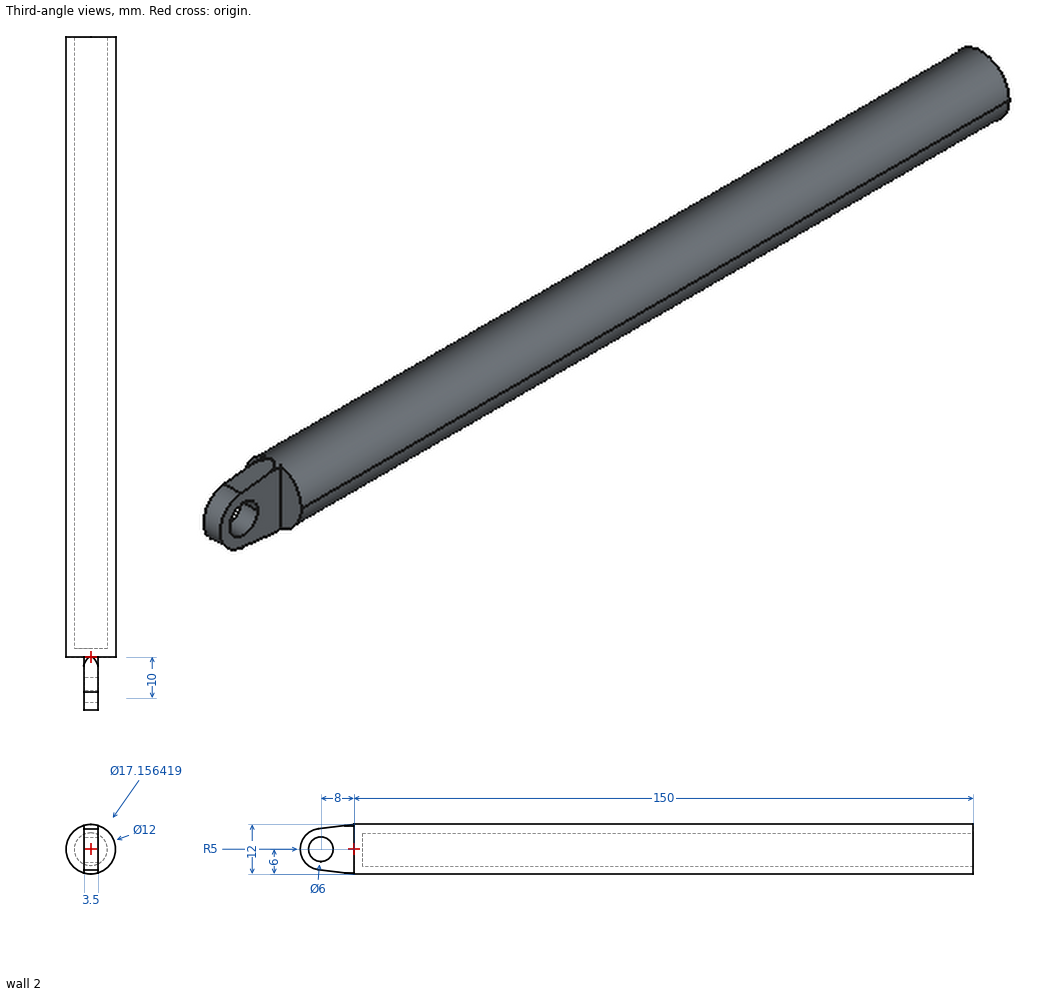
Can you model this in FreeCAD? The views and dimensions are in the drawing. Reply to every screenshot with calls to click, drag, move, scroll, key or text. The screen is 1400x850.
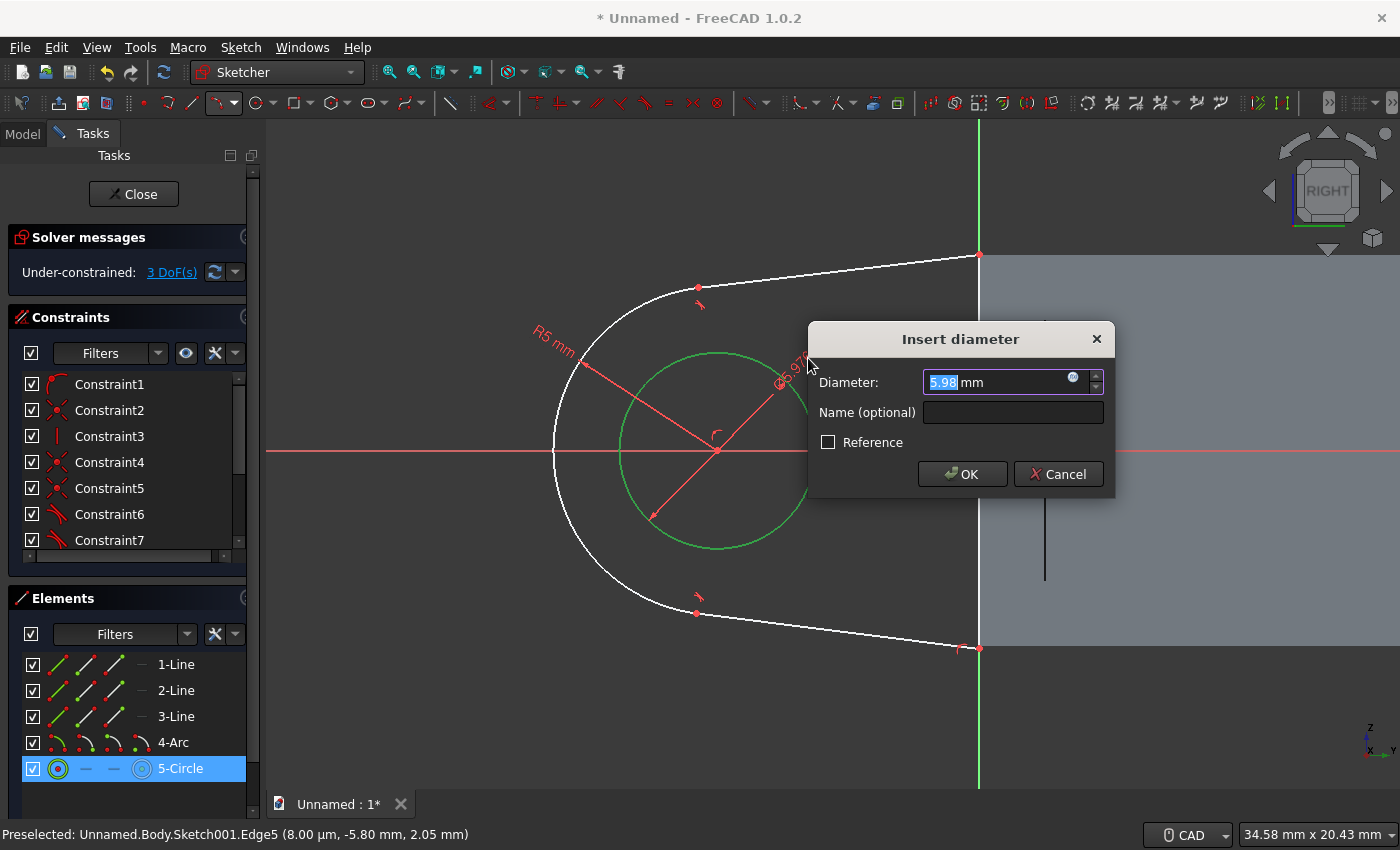
text(6)
key(Return)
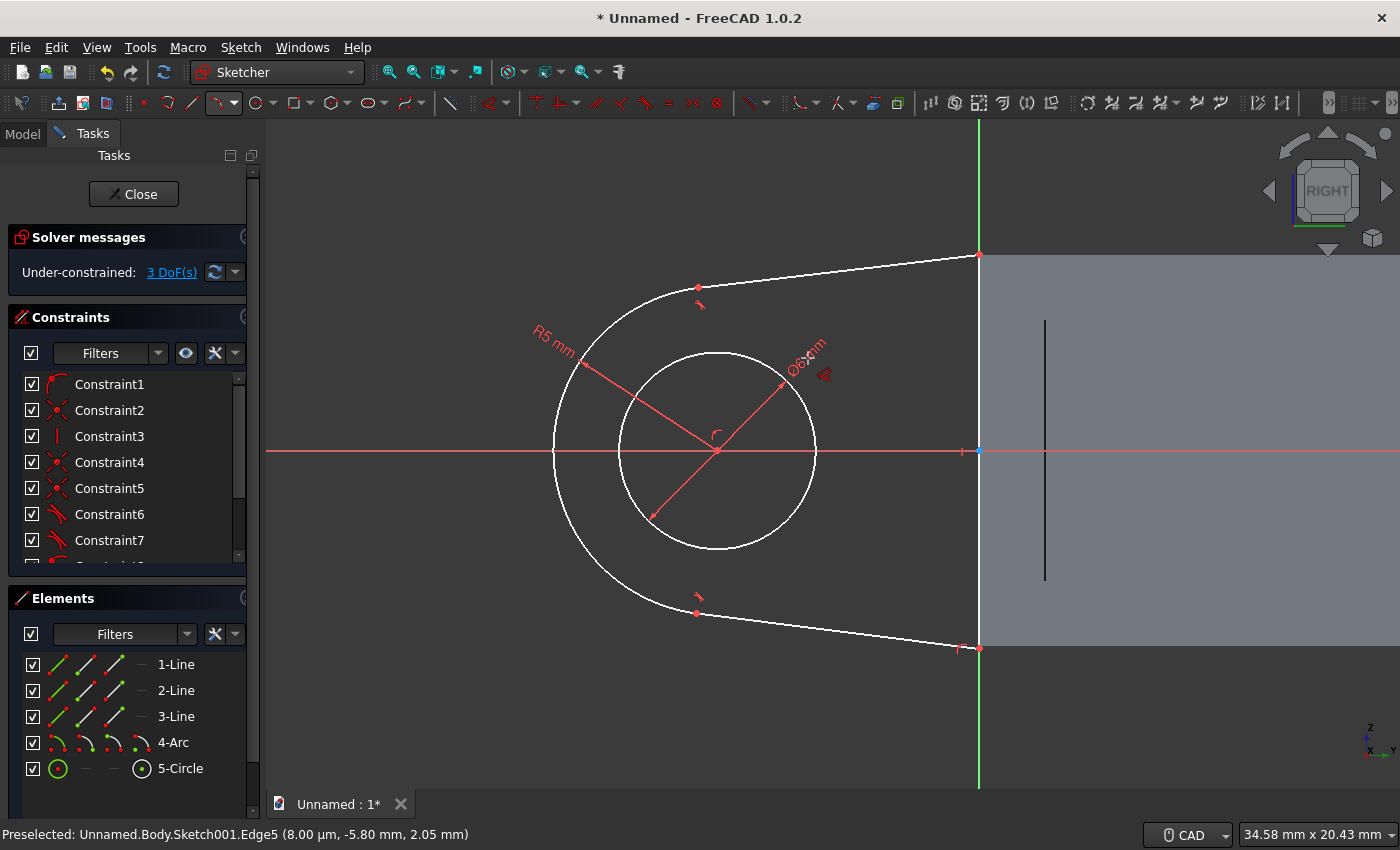
click(717, 451)
click(848, 485)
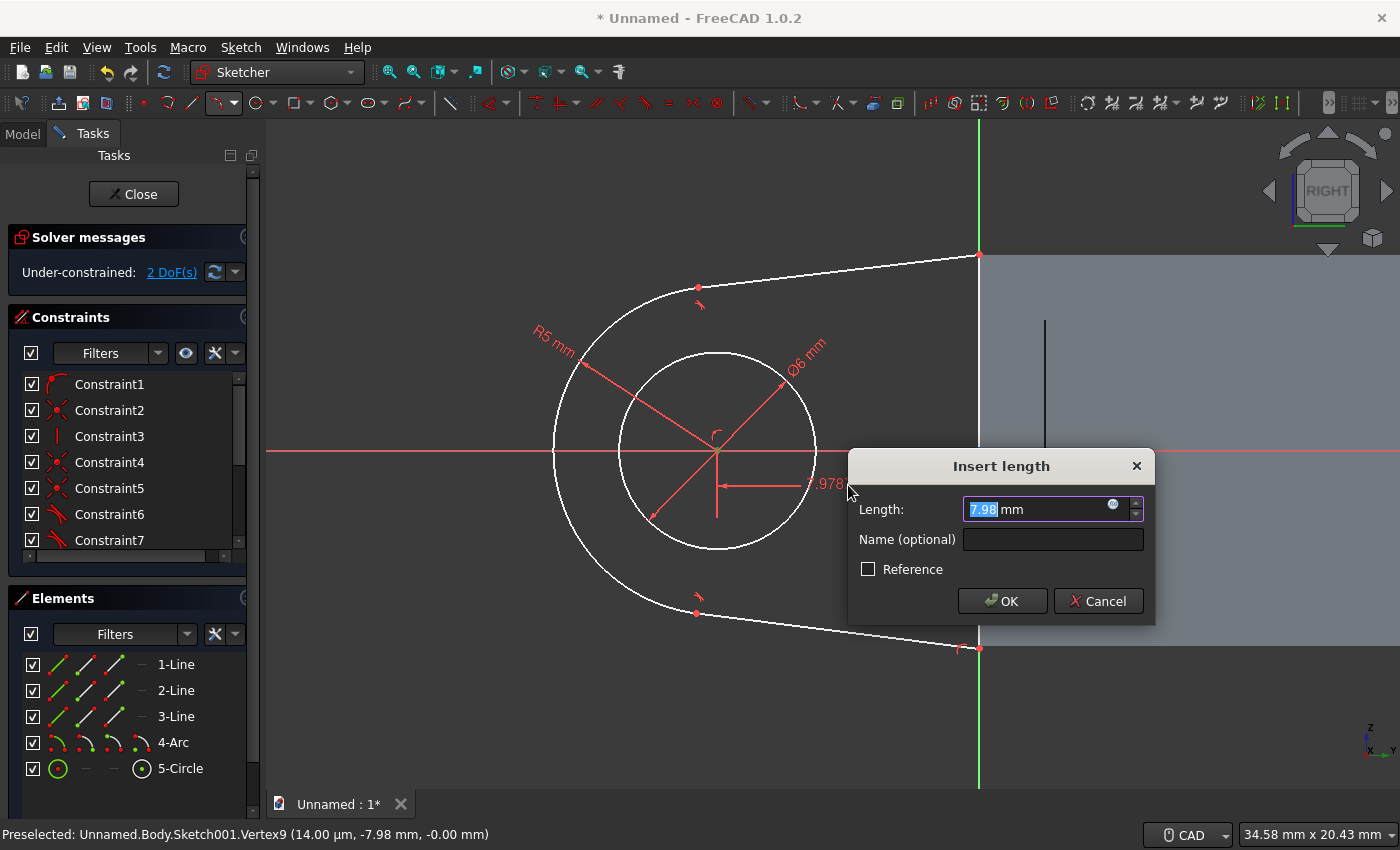
text(8)
key(Return)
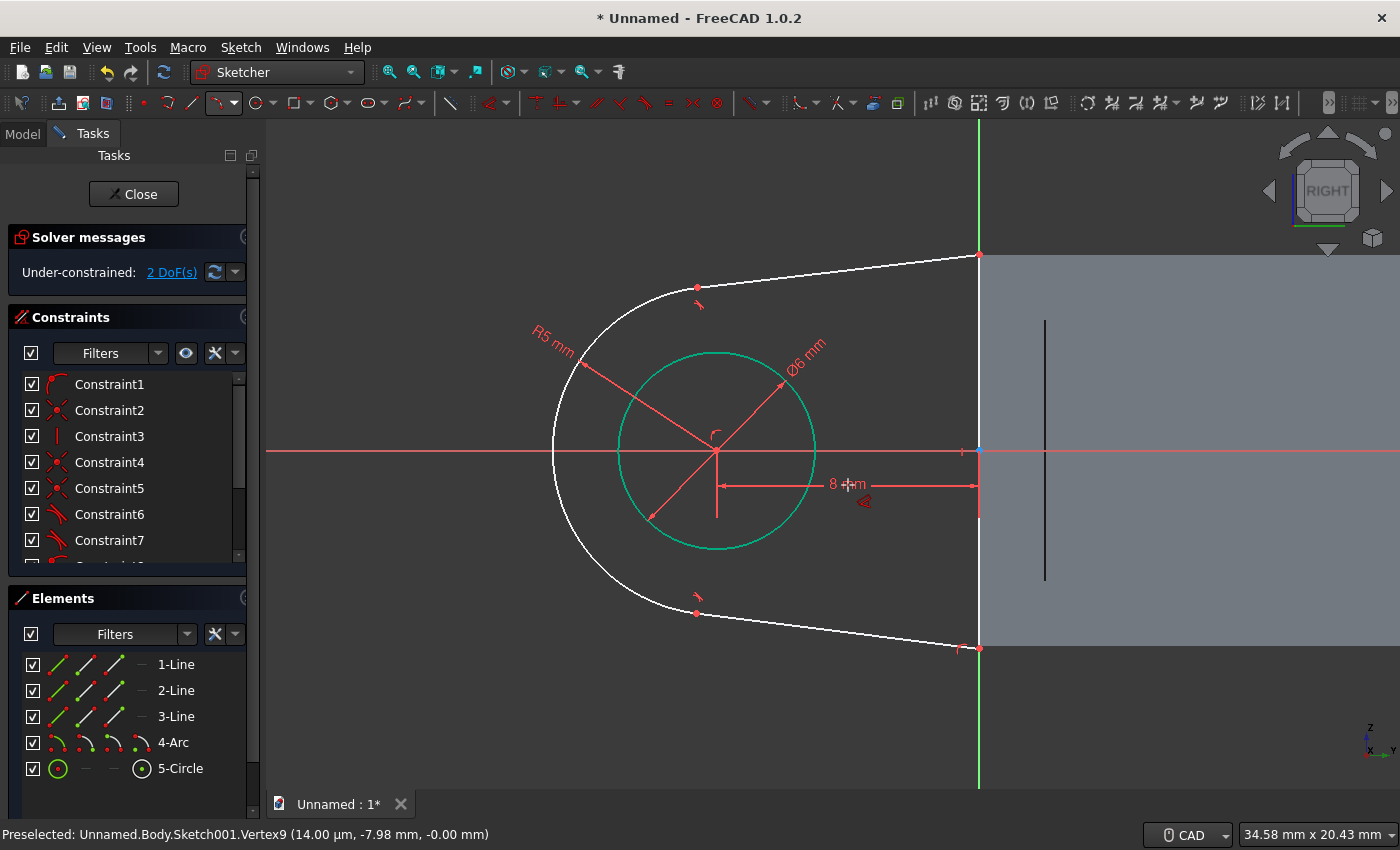
click(979, 531)
click(1013, 361)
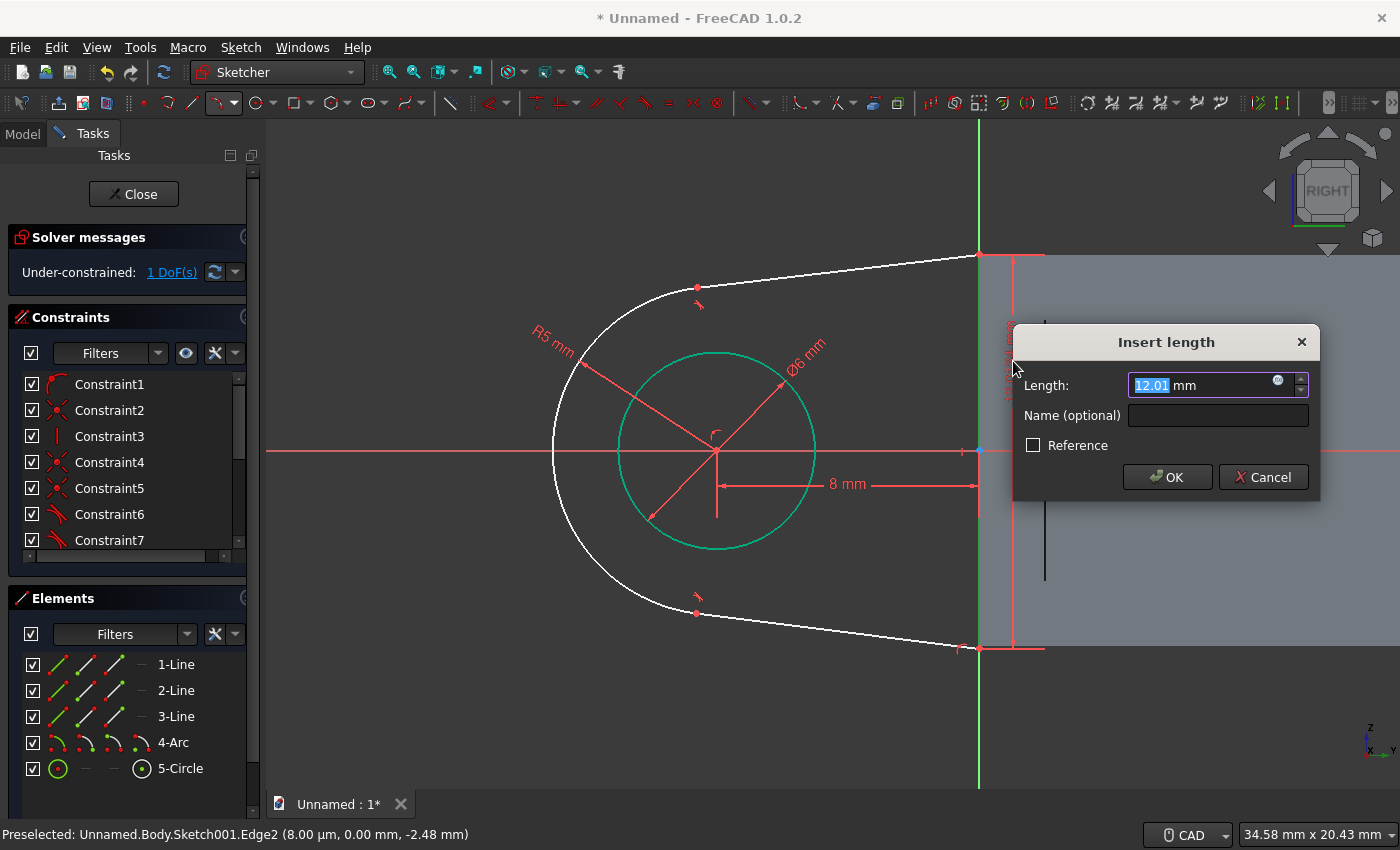
text(12)
key(Return)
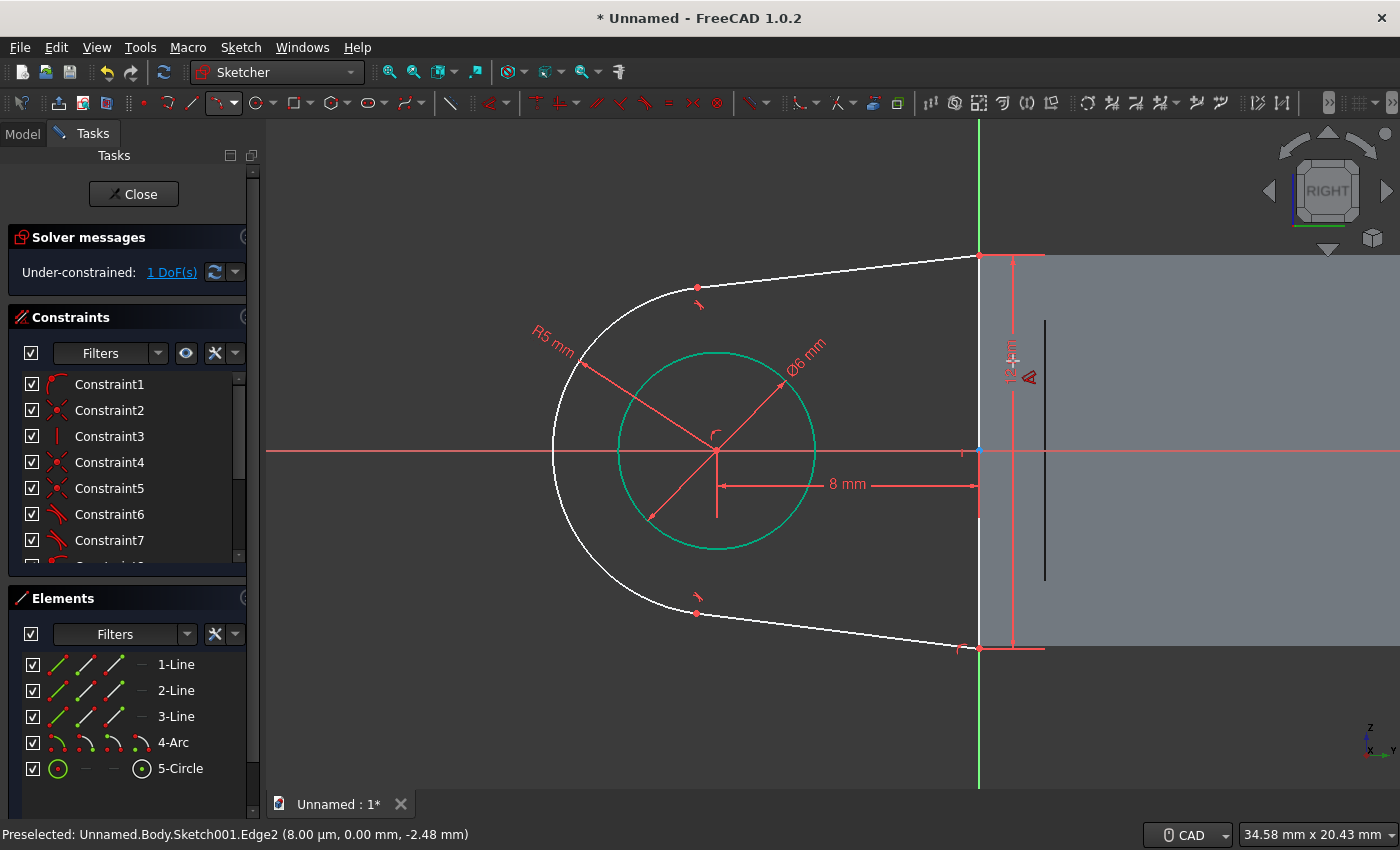
click(979, 649)
click(1013, 550)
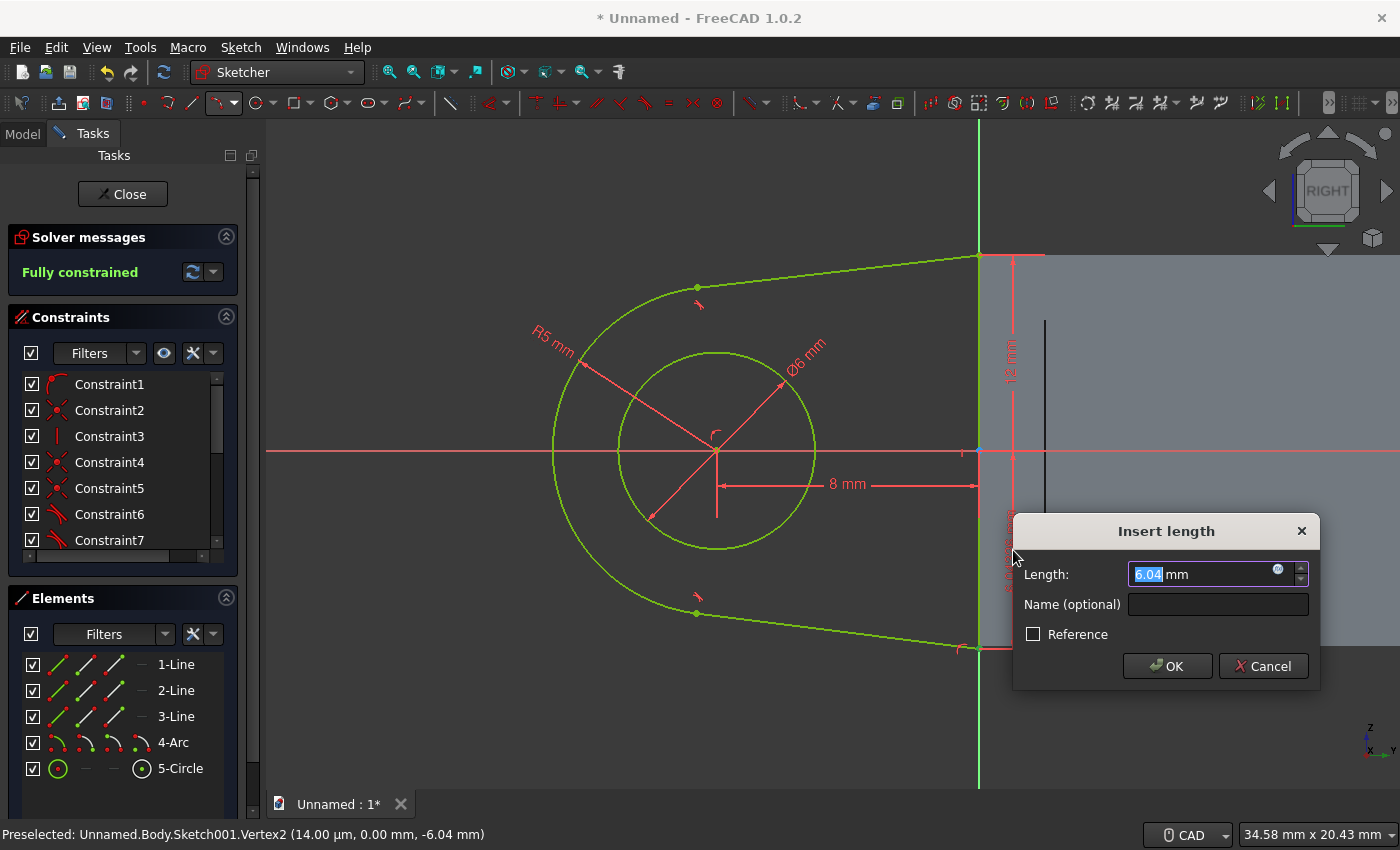
text(6)
key(Return)
key(Escape)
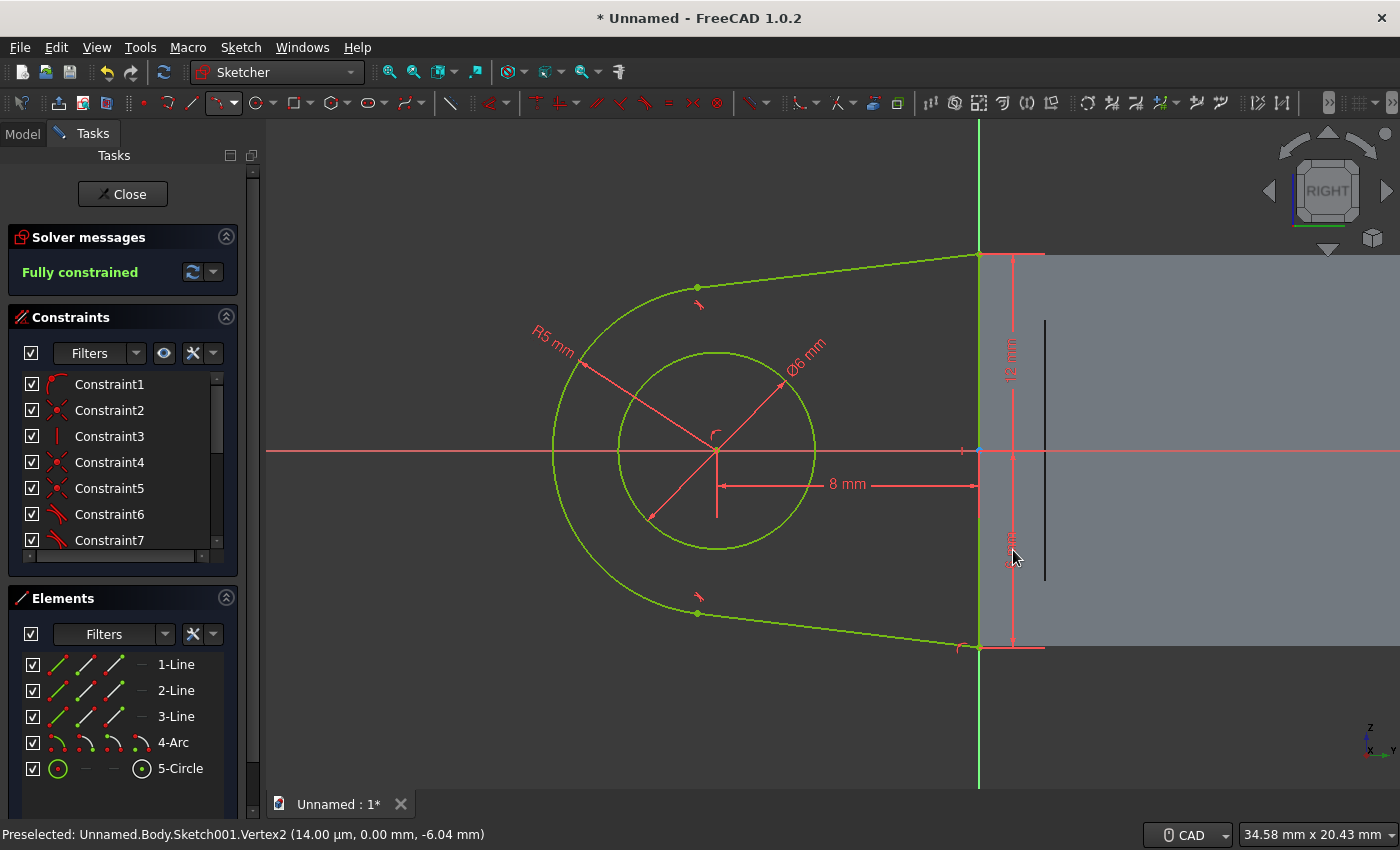
click(123, 194)